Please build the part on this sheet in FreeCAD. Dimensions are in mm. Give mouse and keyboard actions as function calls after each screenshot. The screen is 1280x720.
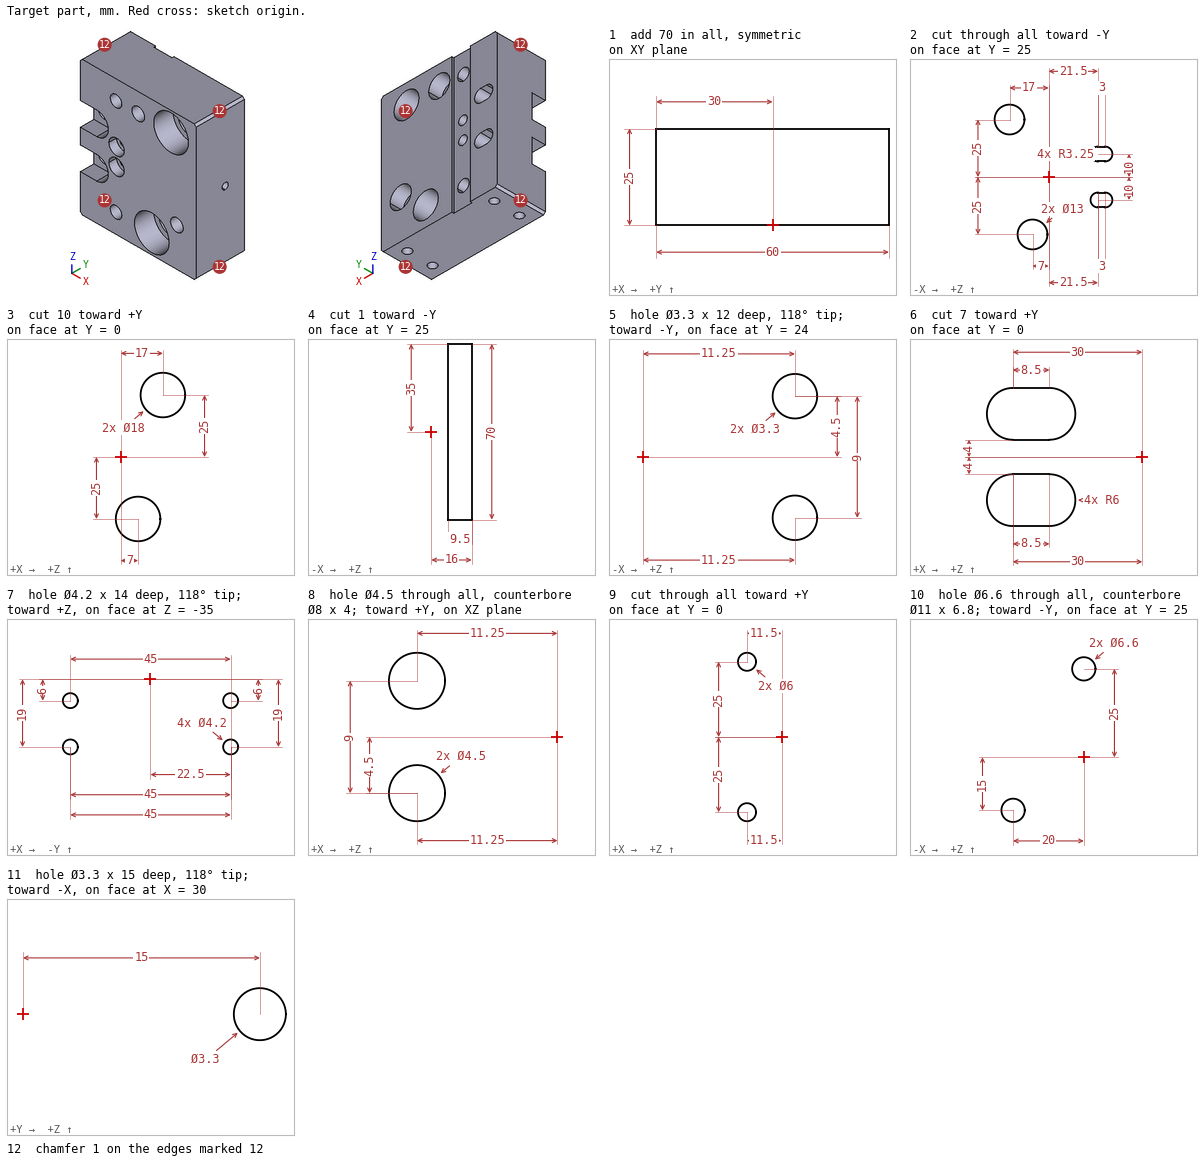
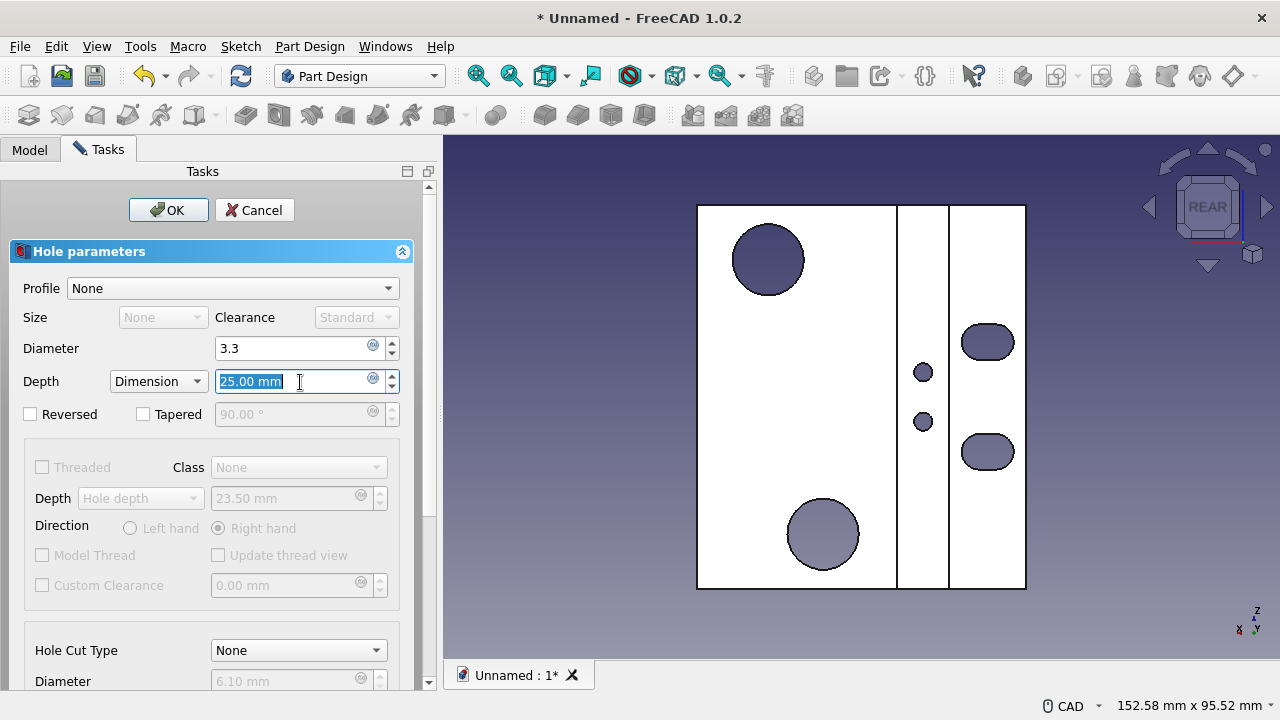
text(12)
key(Tab)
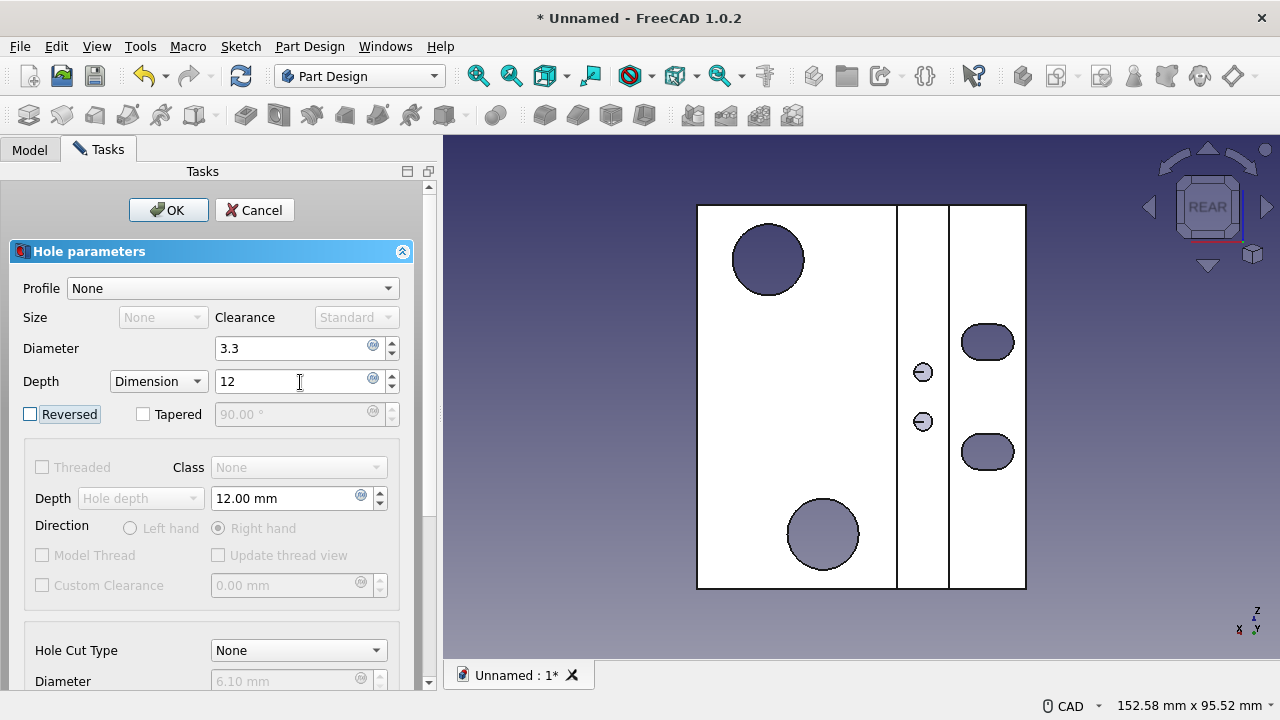
click(169, 210)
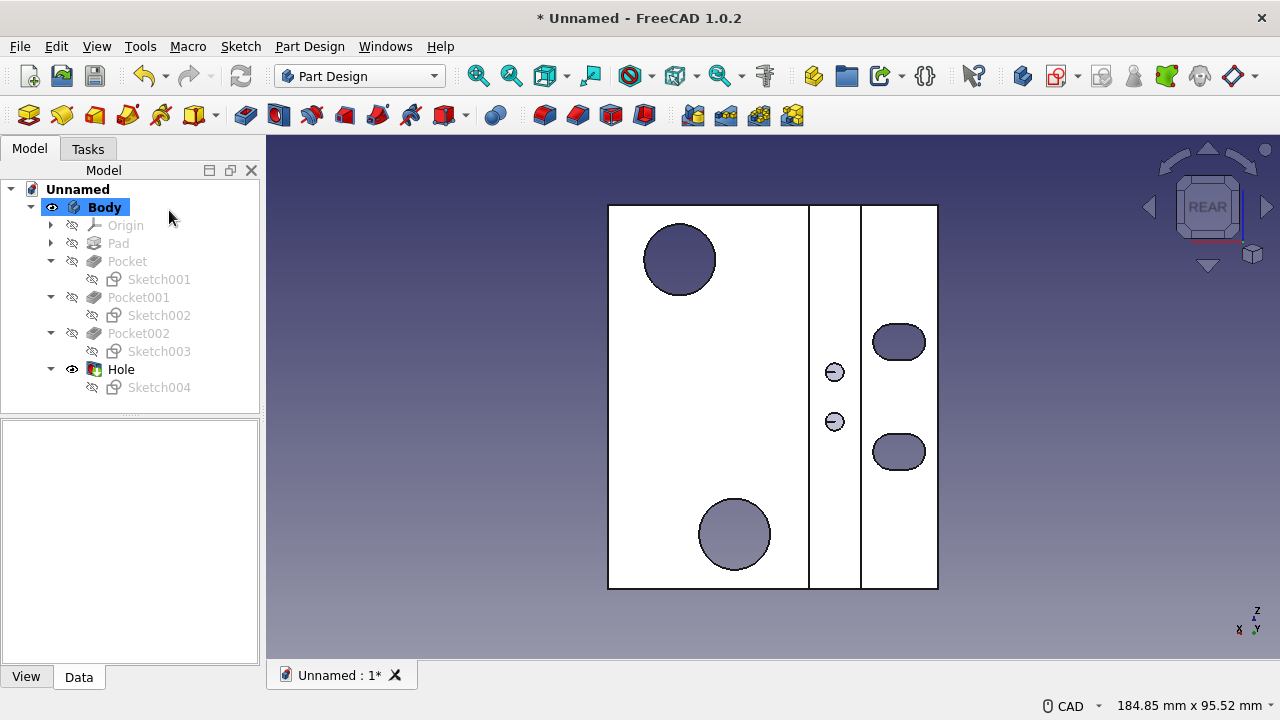
key(0)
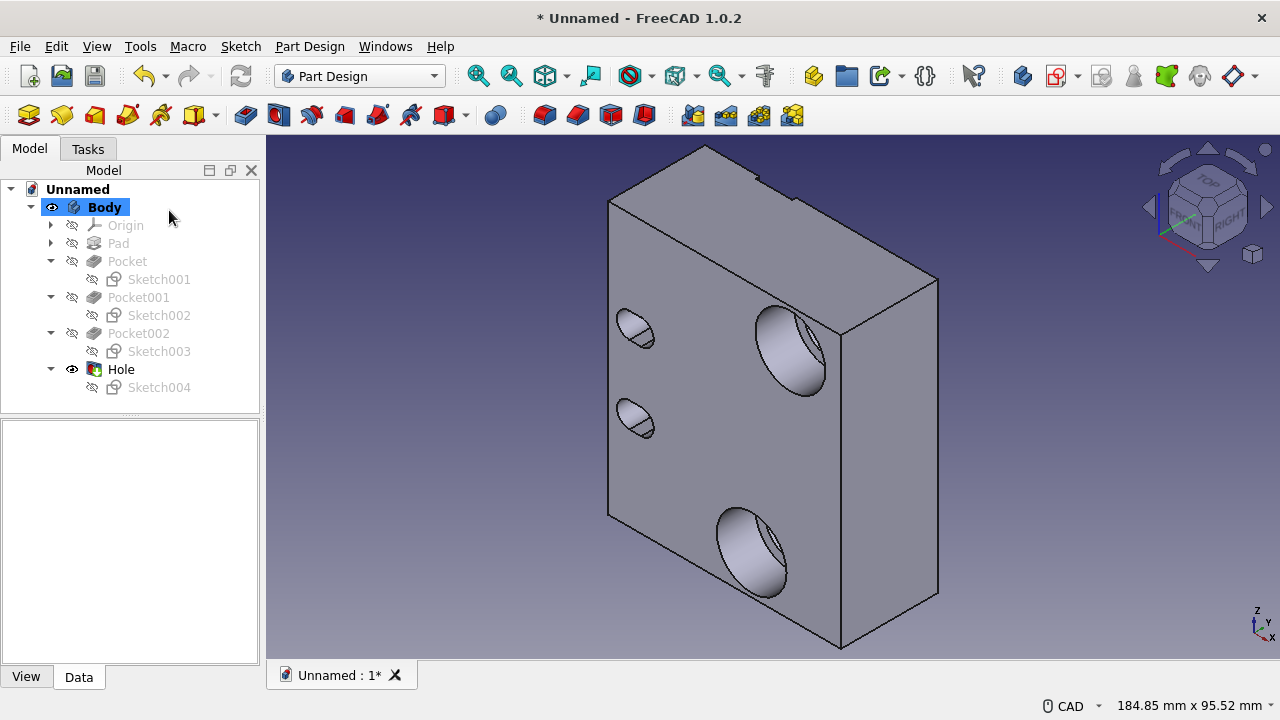
click(725, 424)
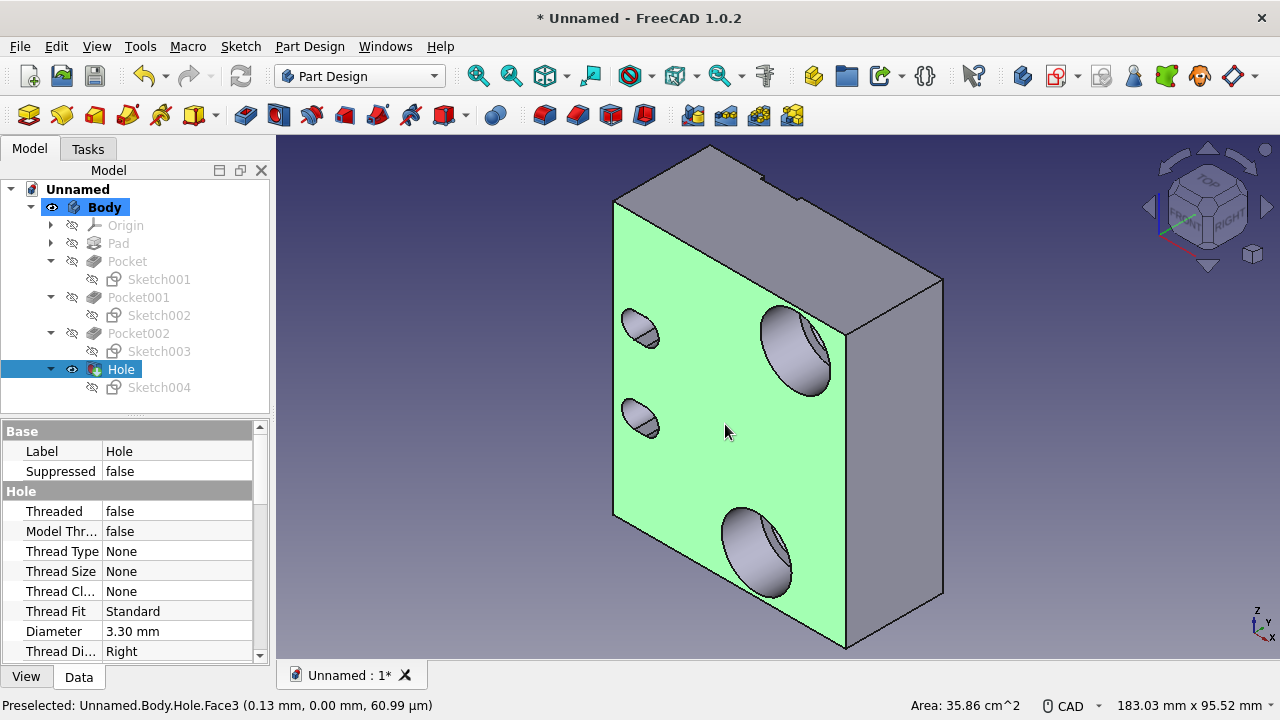
click(1056, 76)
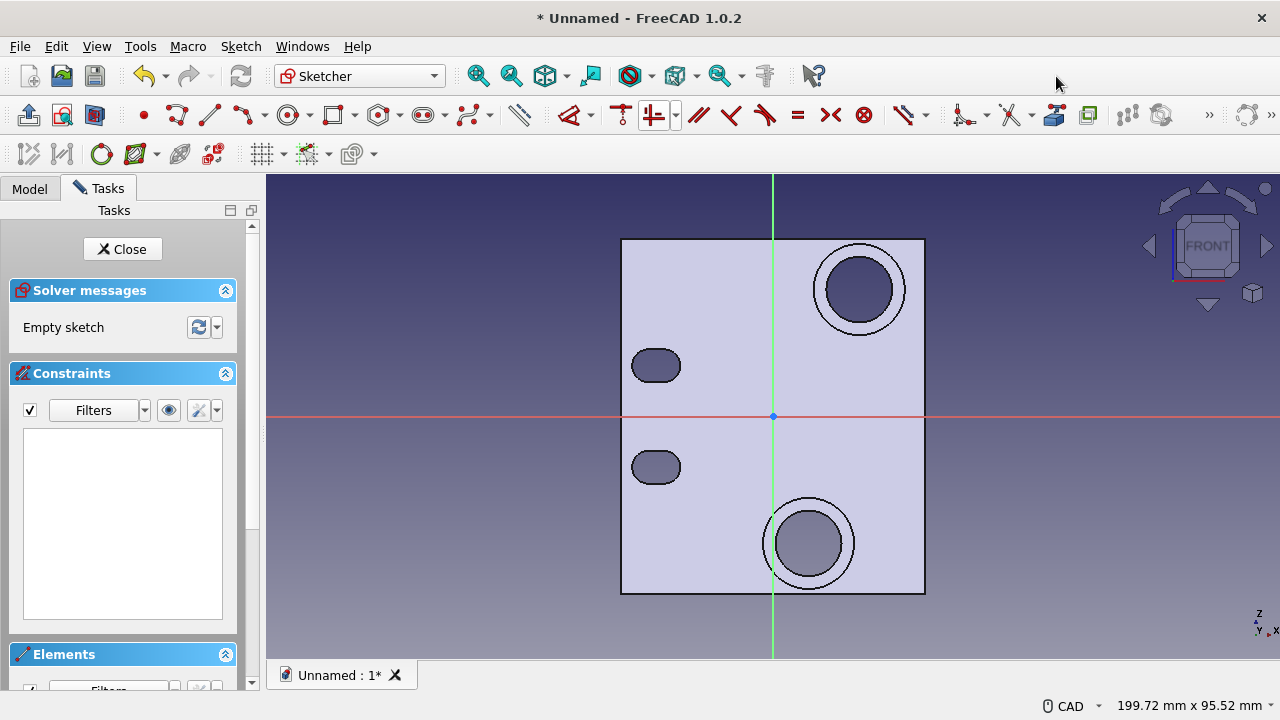
scroll(654, 417, up, 3)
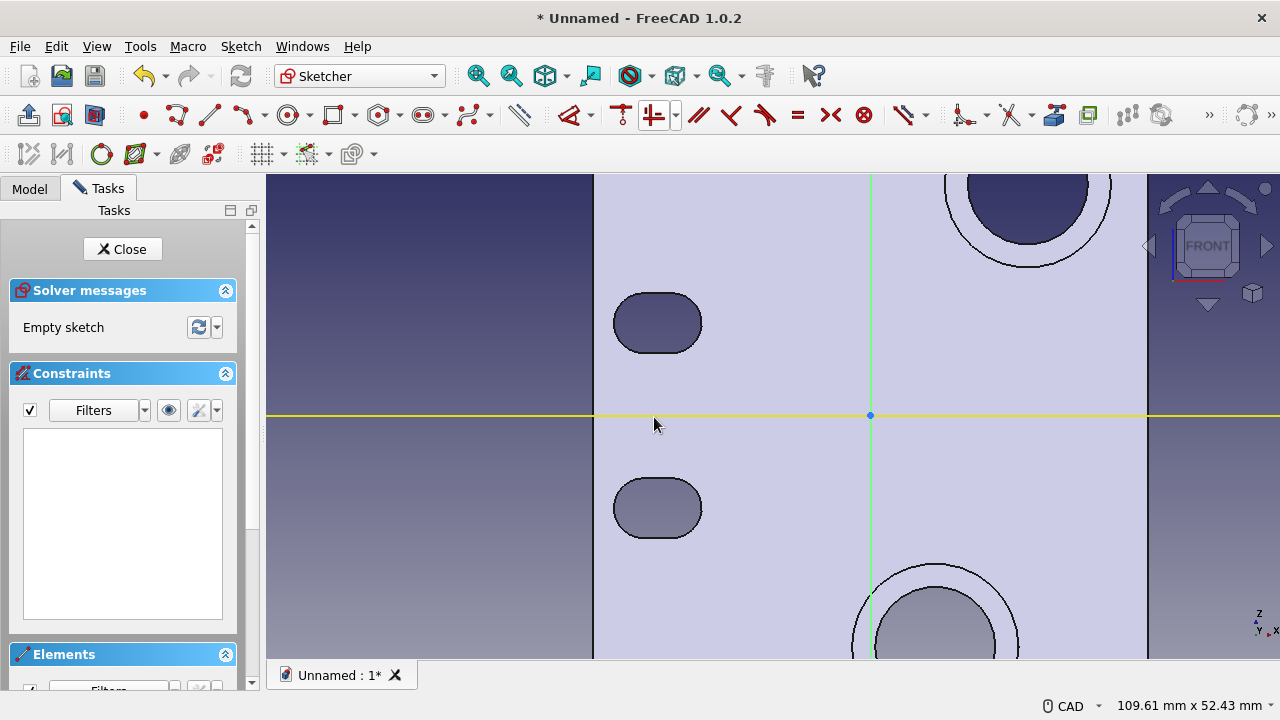
key(g)
key(s)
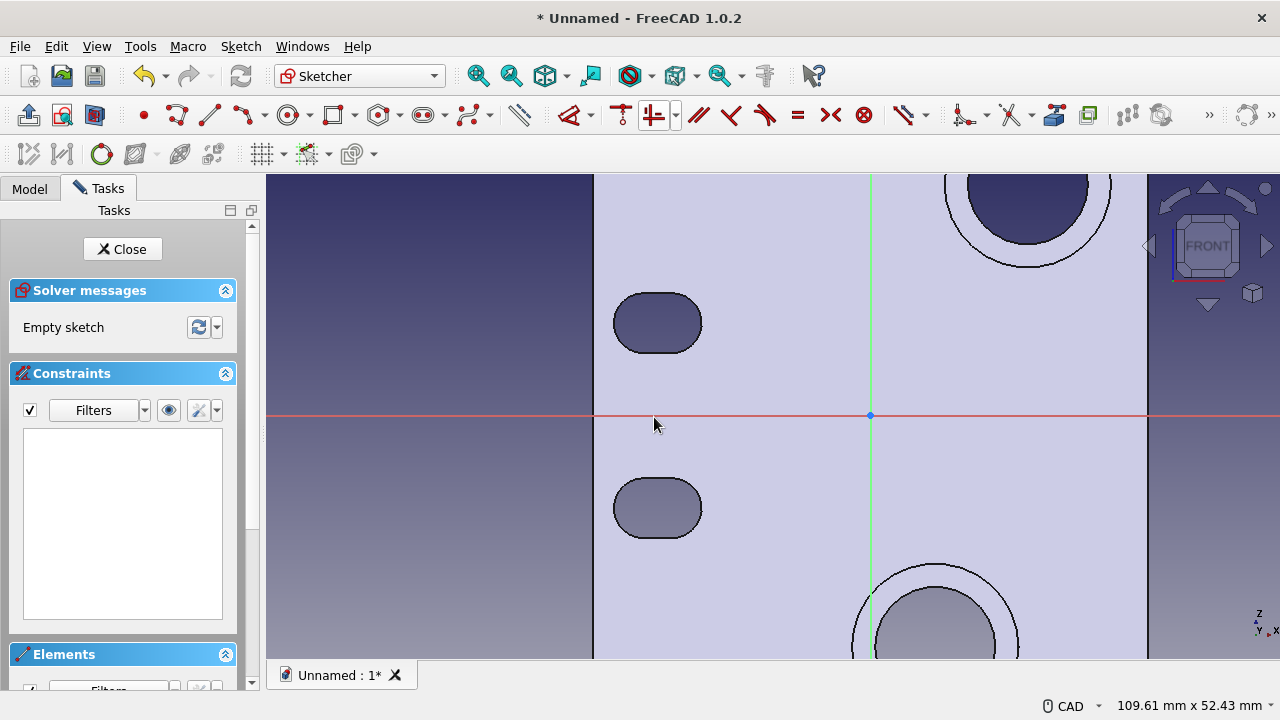
click(593, 508)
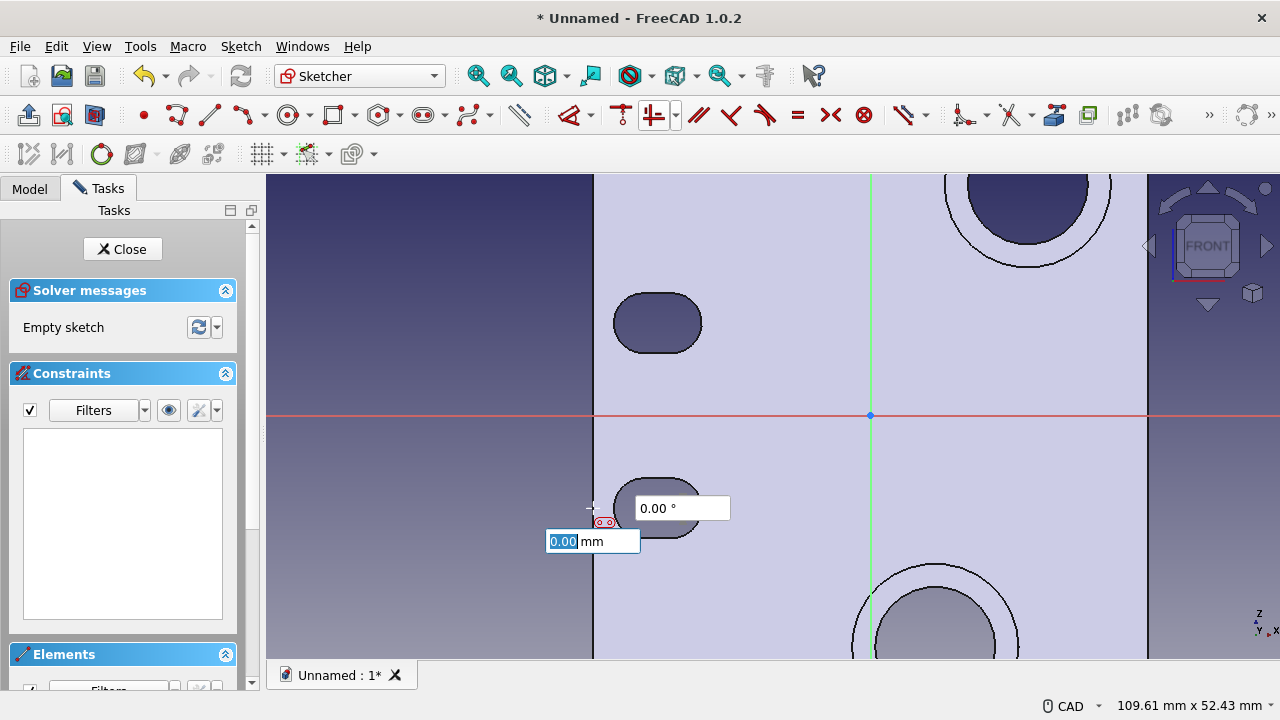
click(672, 508)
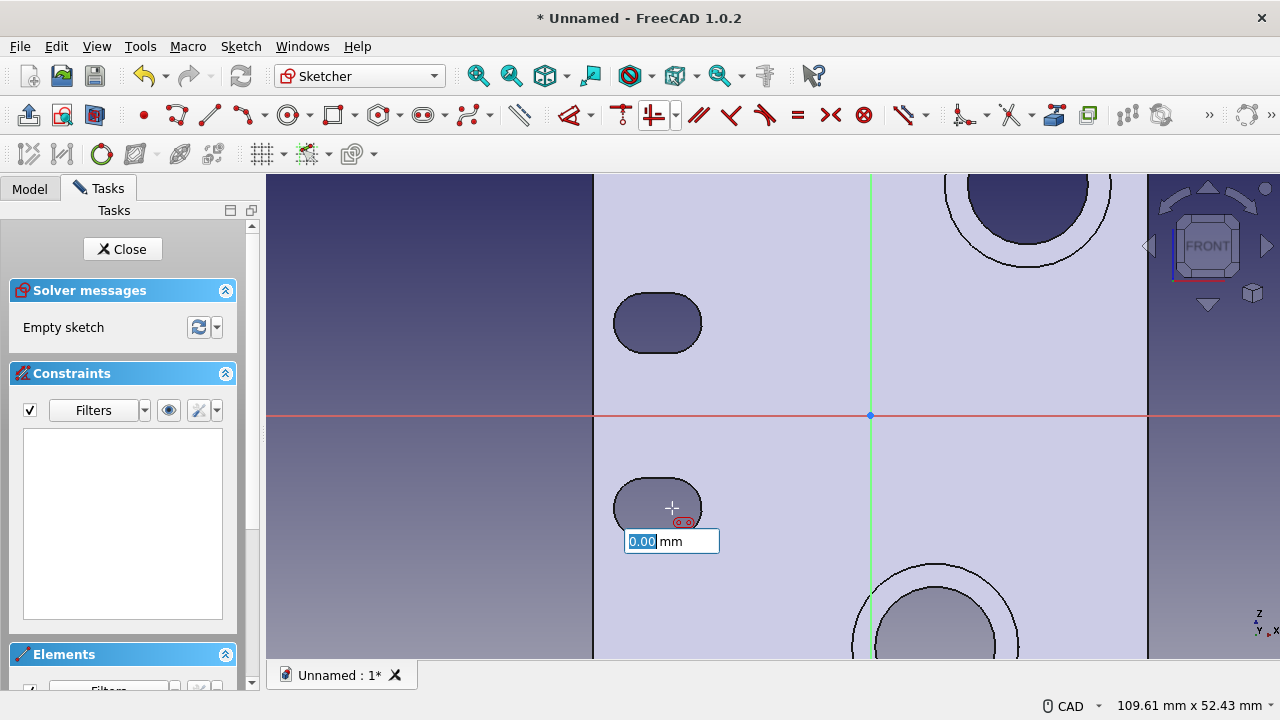
click(632, 564)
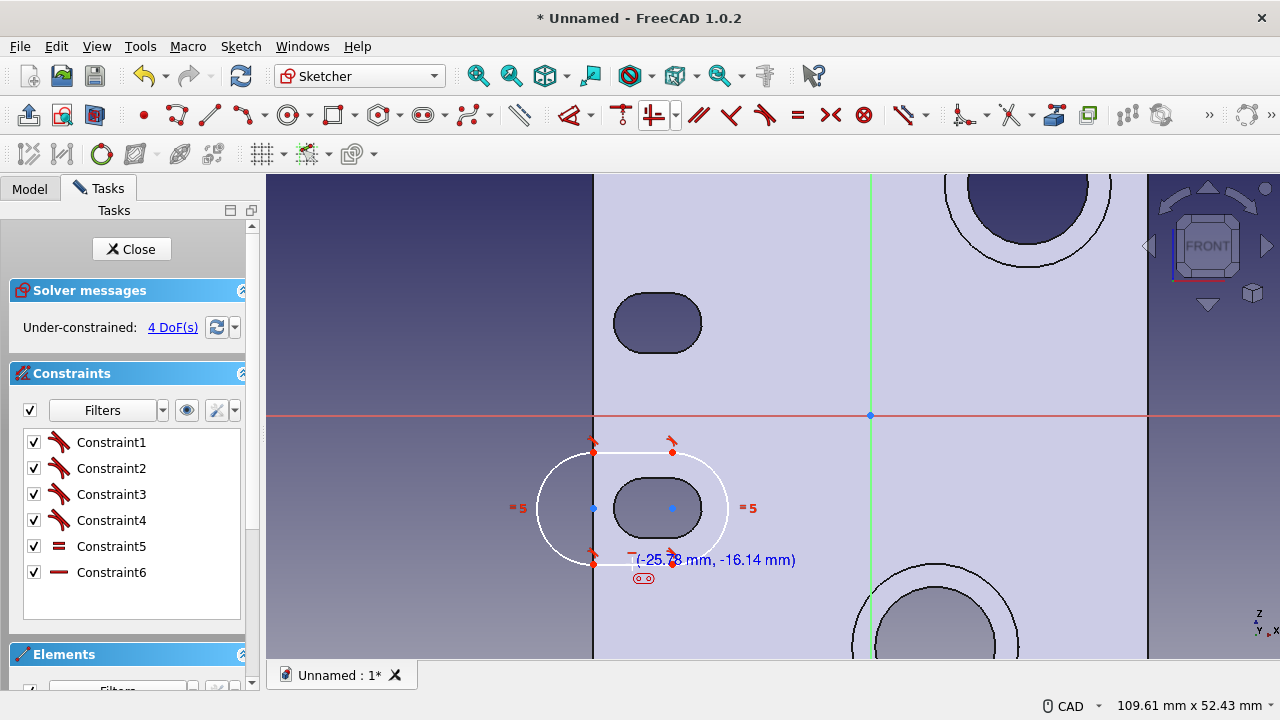
click(593, 323)